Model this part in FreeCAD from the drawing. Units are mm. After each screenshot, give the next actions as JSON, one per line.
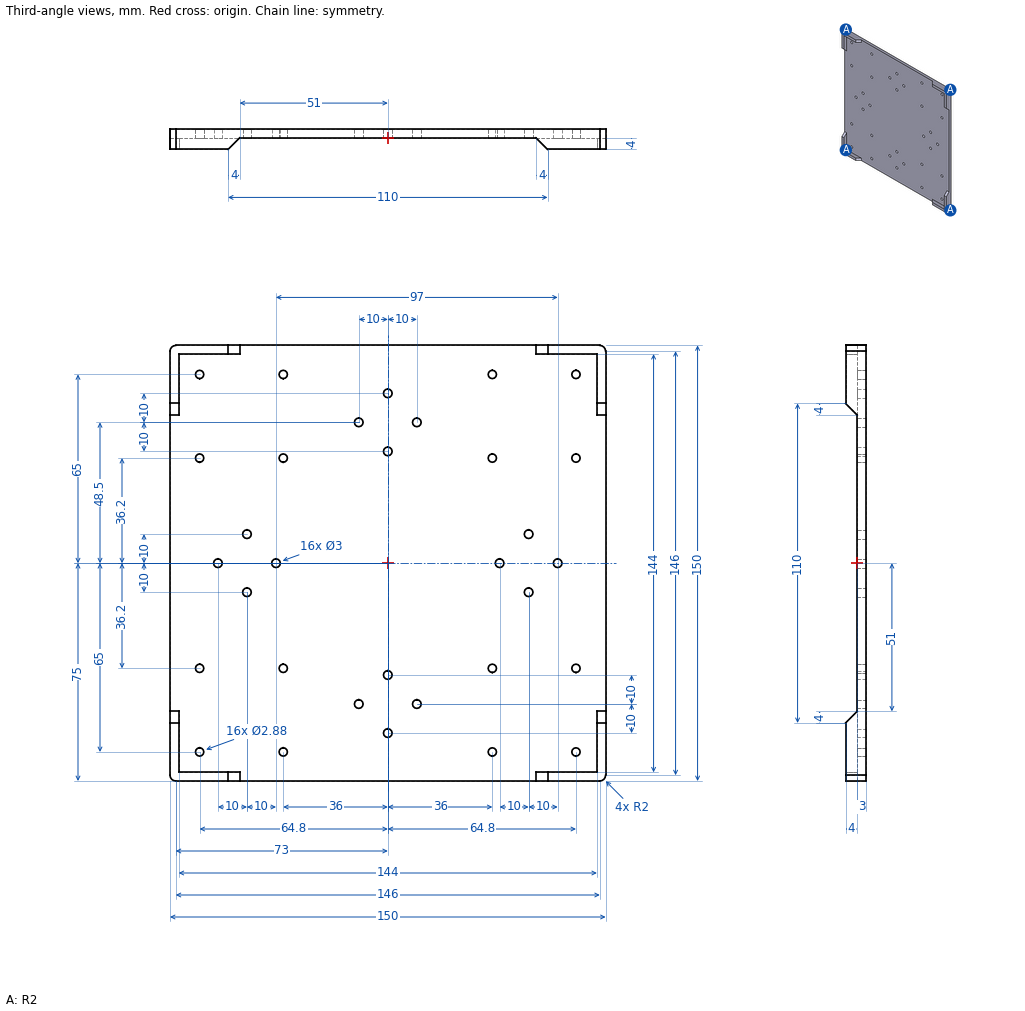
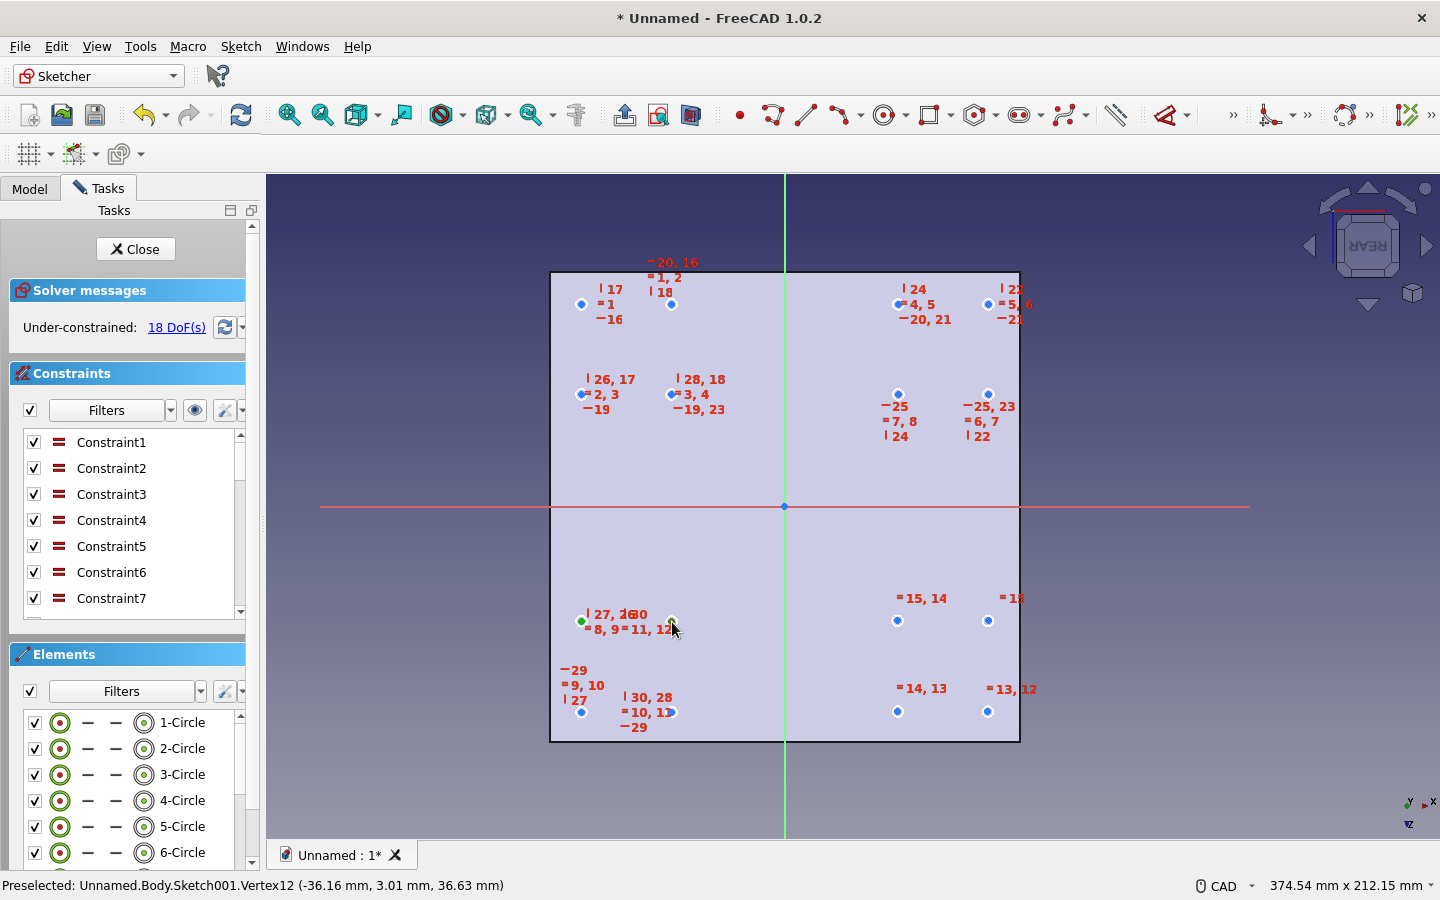
{"action": "key", "text": "h"}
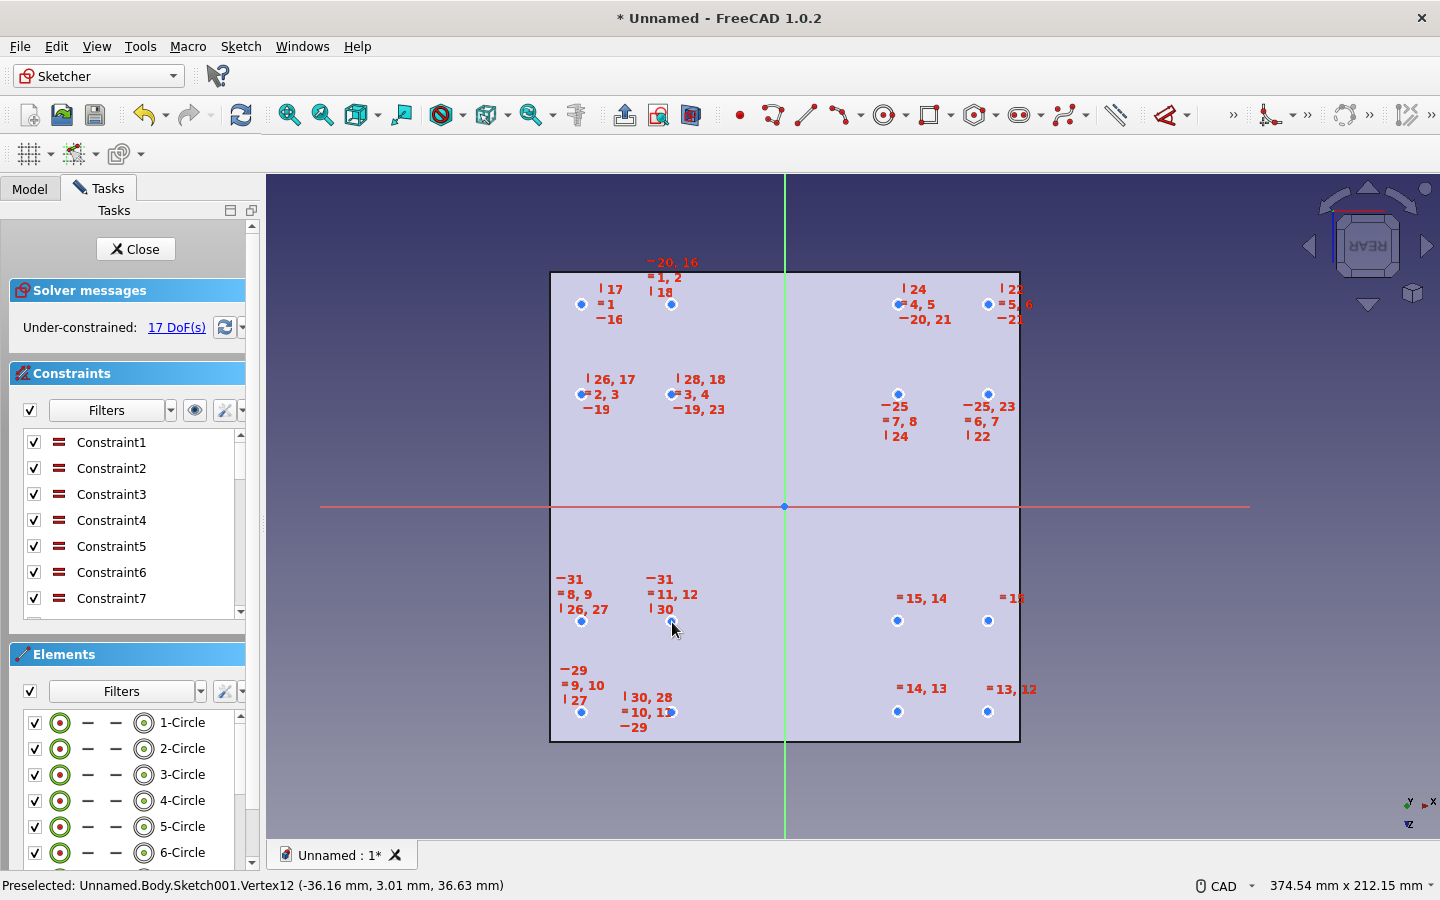
{"action": "left_click", "coordinate": [988, 394]}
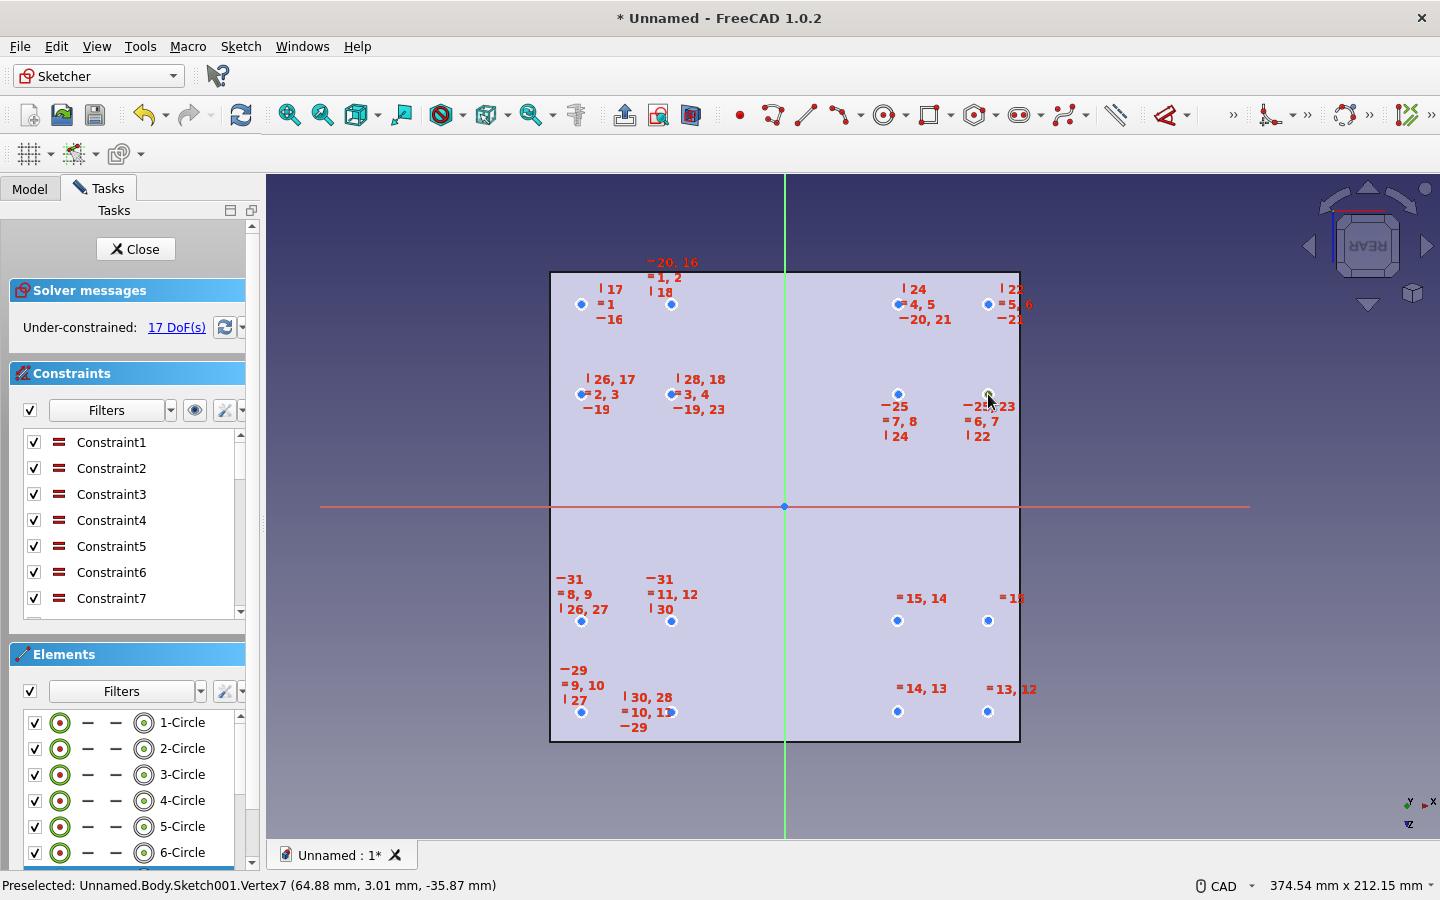
{"action": "left_click", "coordinate": [988, 712]}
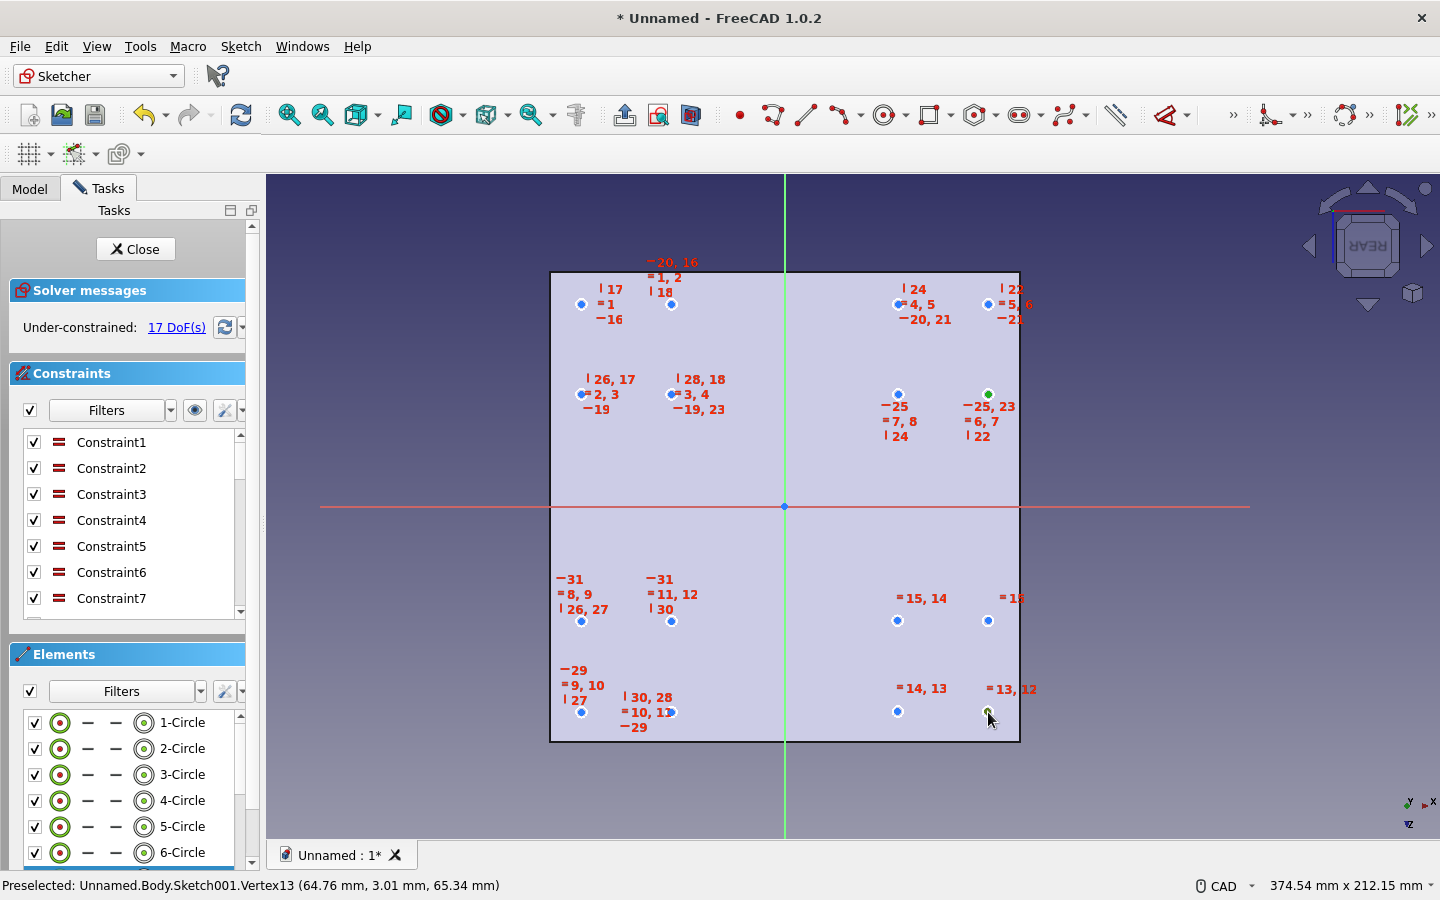
{"action": "key", "text": "v"}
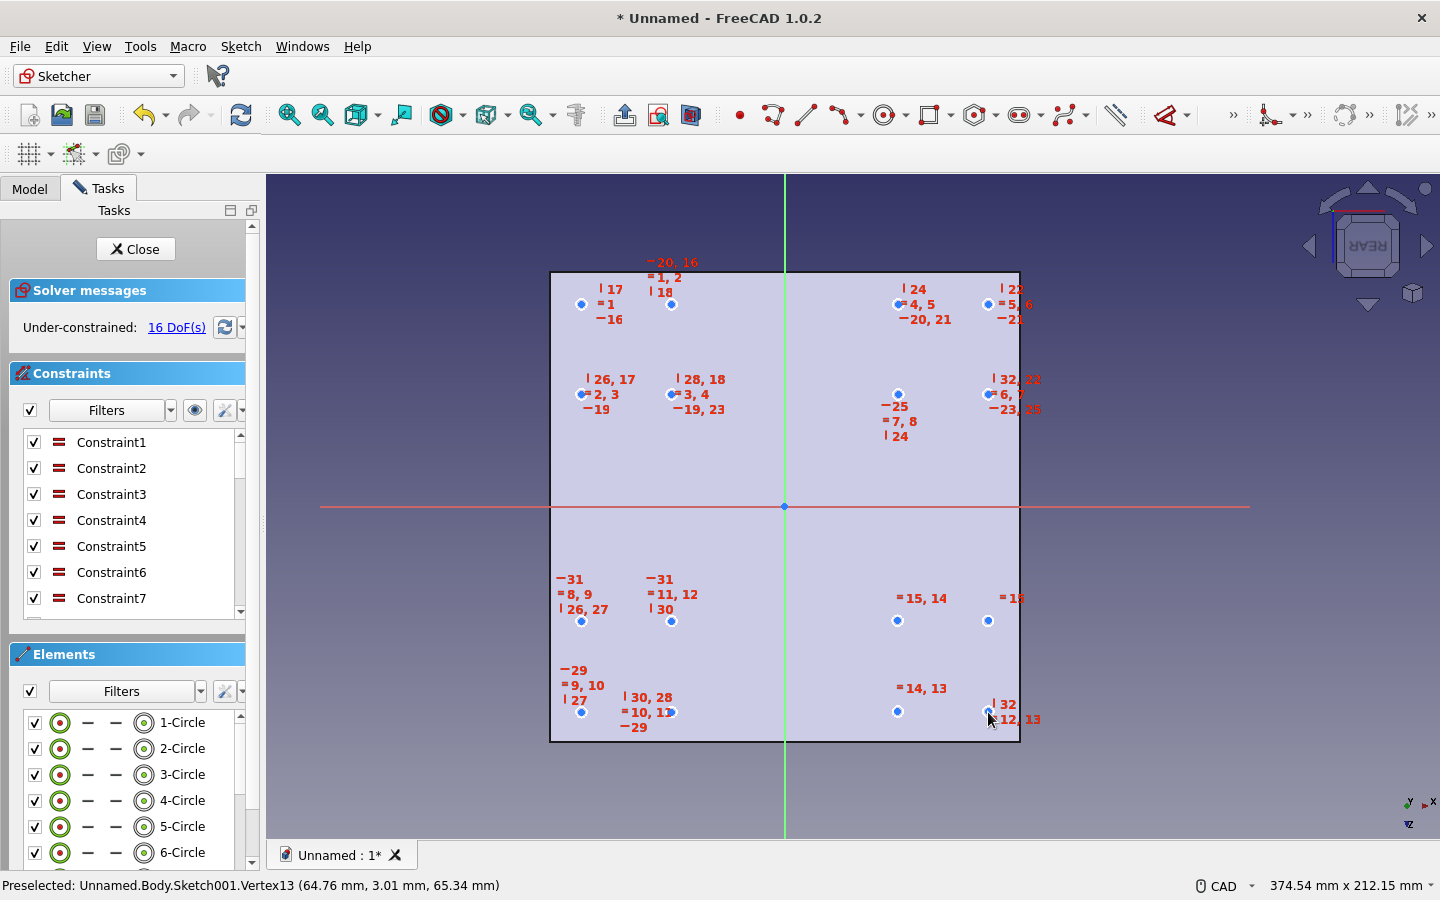
{"action": "left_click", "coordinate": [672, 712]}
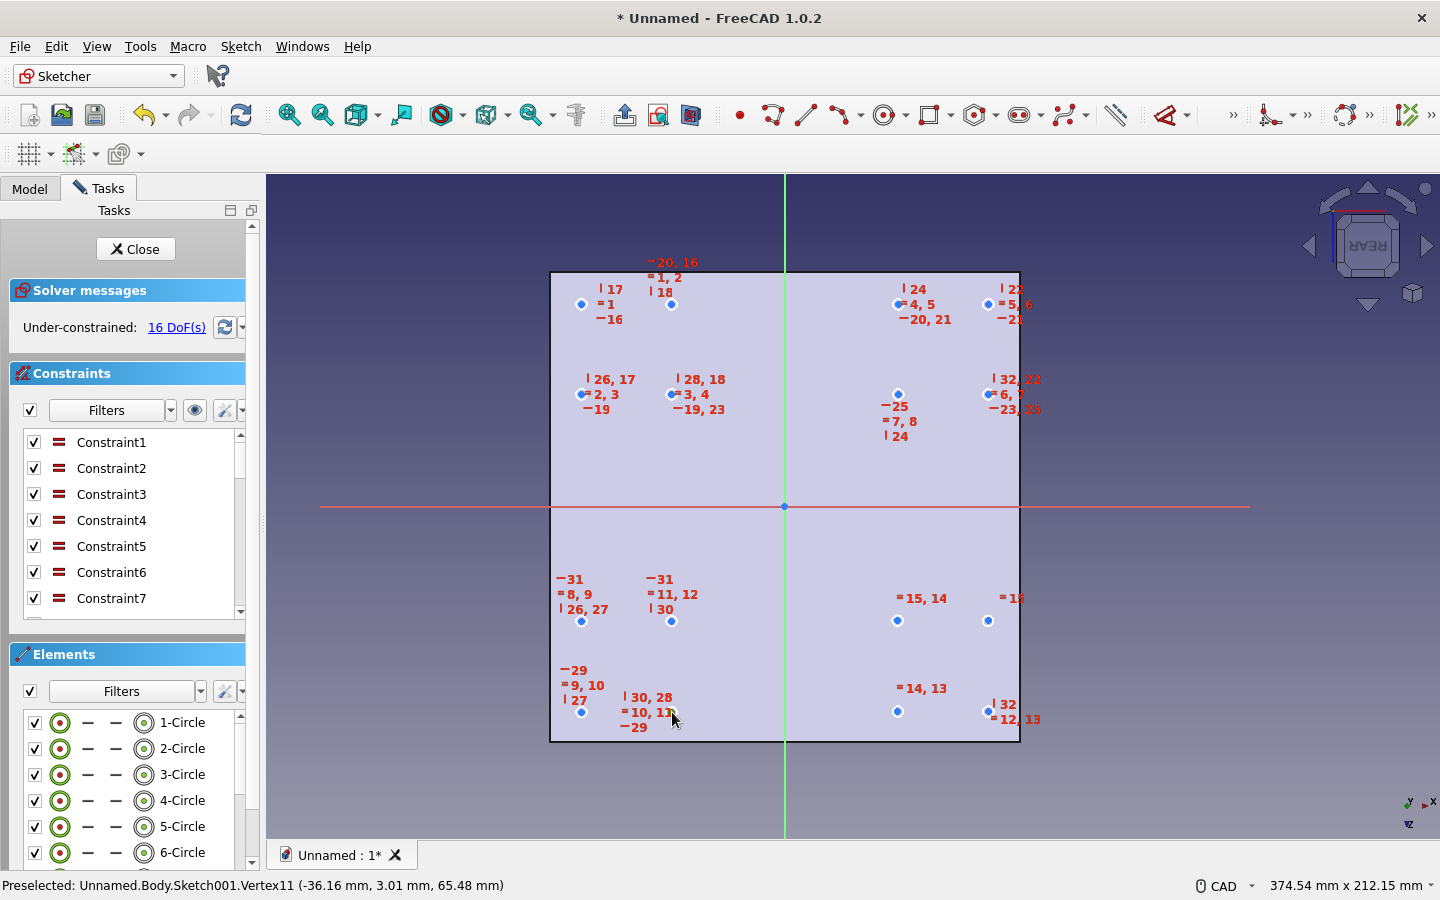
{"action": "left_click", "coordinate": [988, 712]}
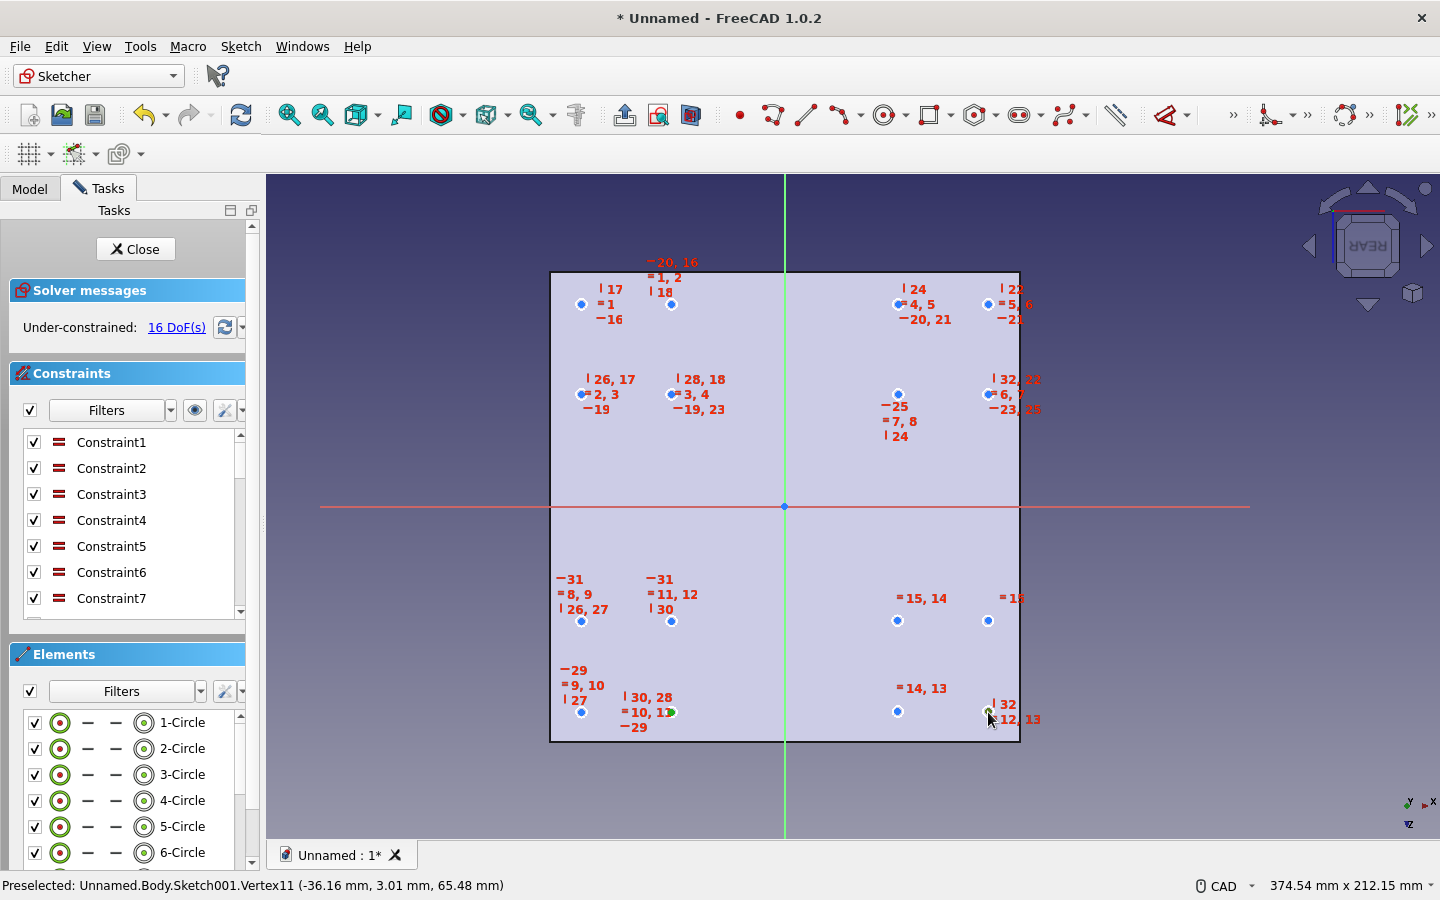
{"action": "key", "text": "h"}